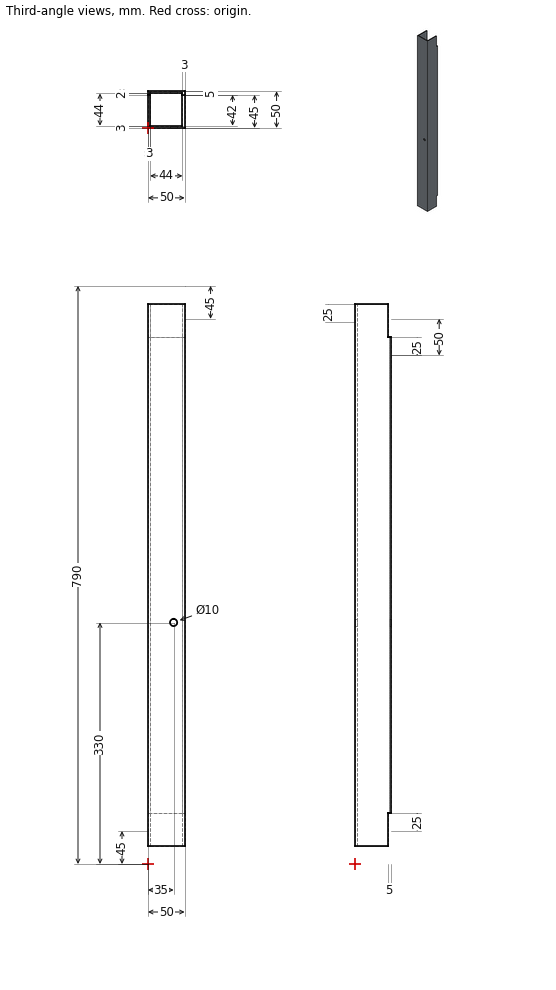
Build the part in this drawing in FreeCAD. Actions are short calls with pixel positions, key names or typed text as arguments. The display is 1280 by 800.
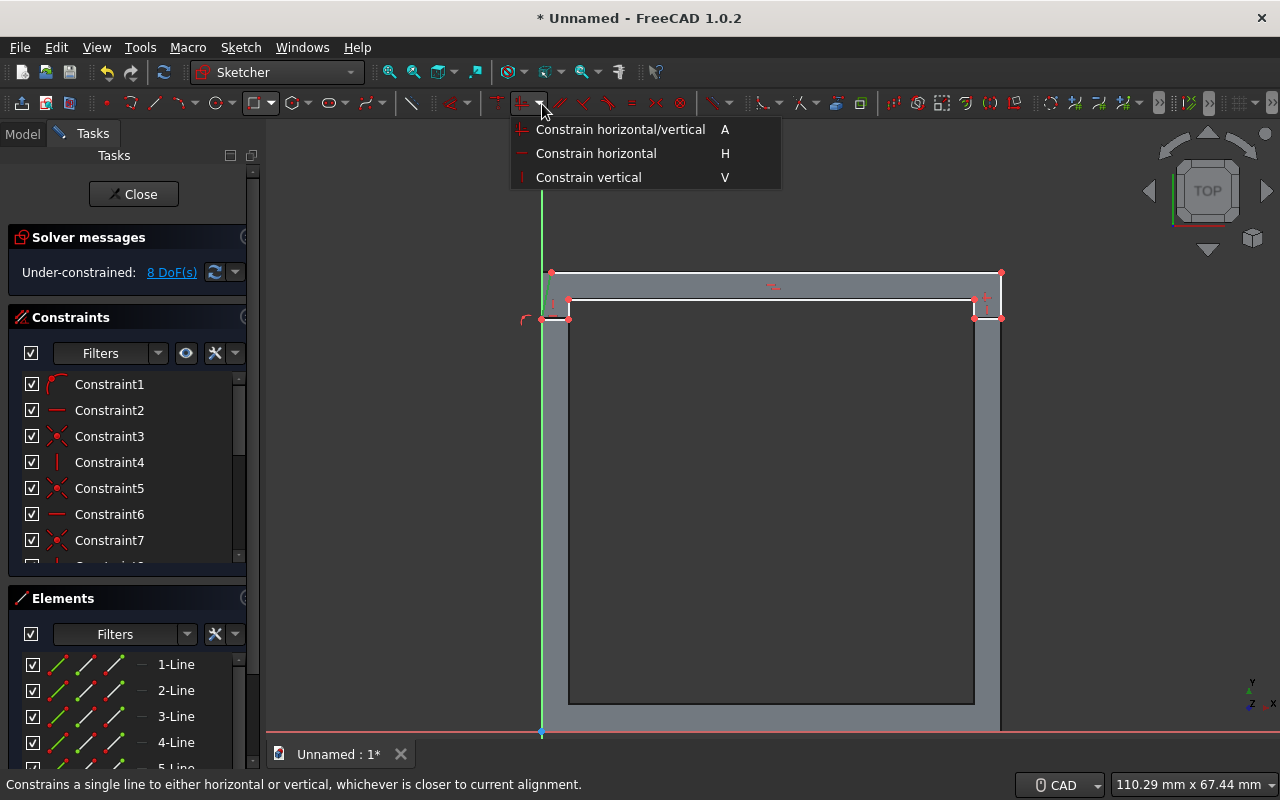
click(646, 177)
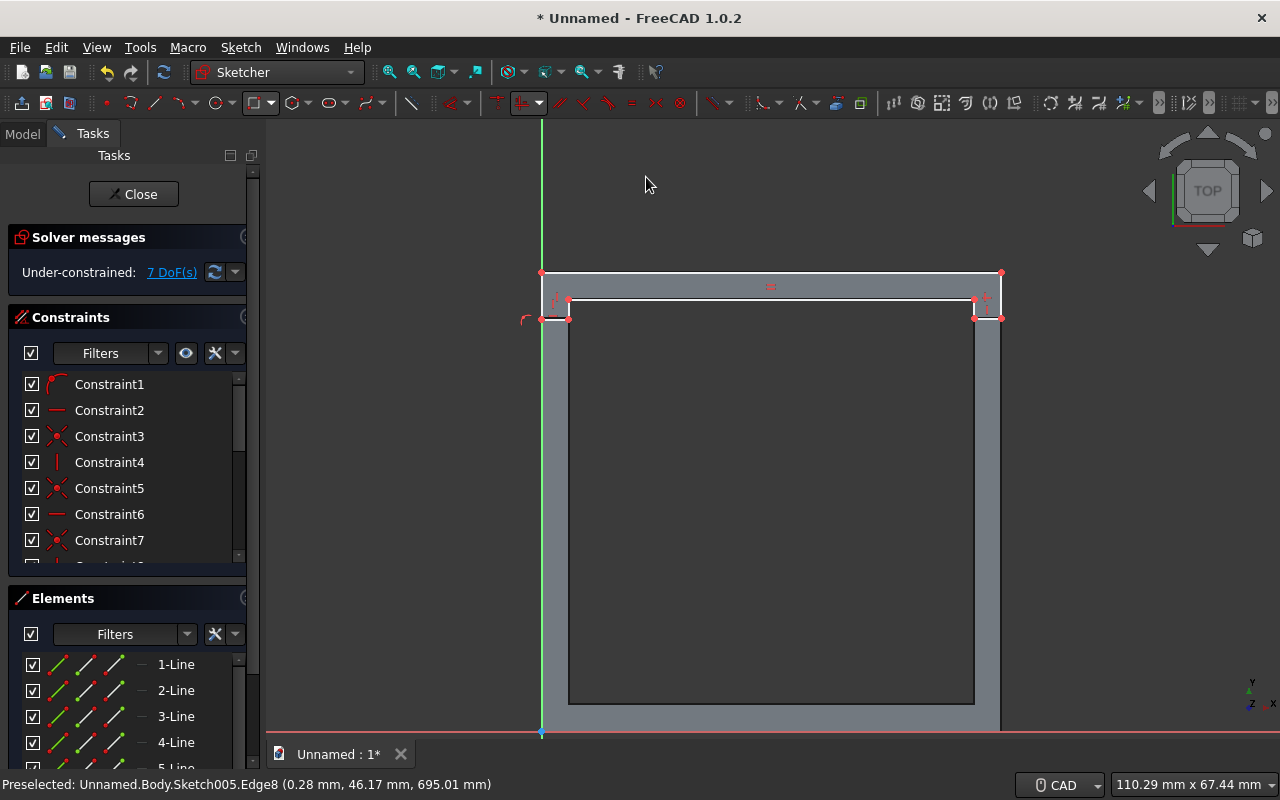
click(450, 104)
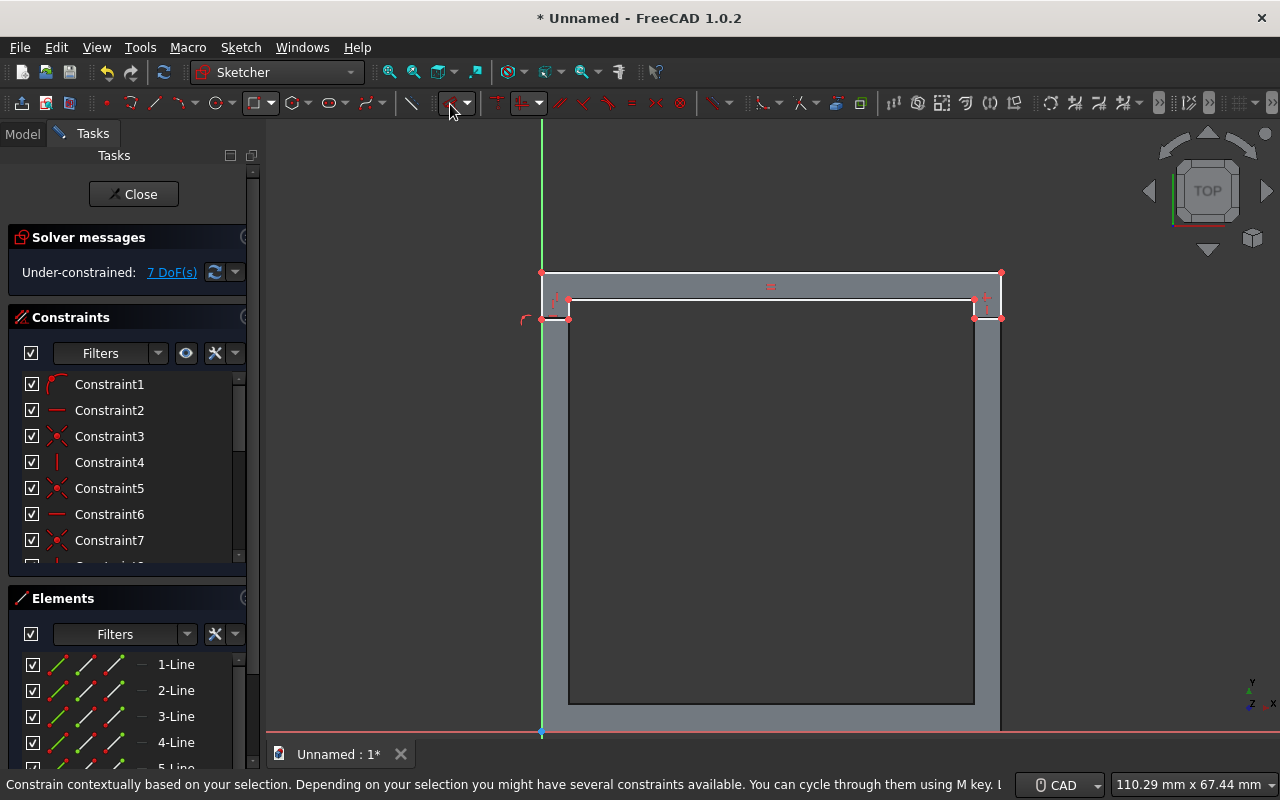
scroll(552, 320, up, 2)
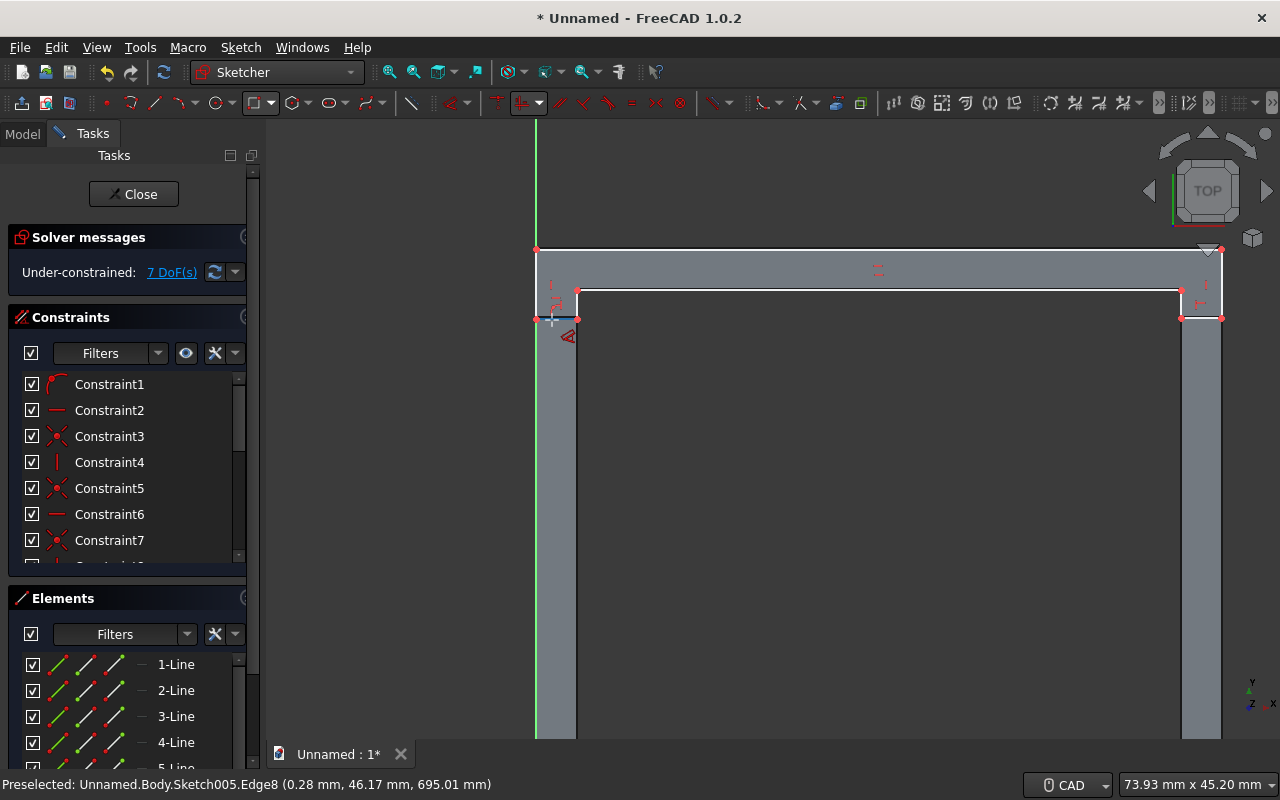
click(553, 319)
click(557, 285)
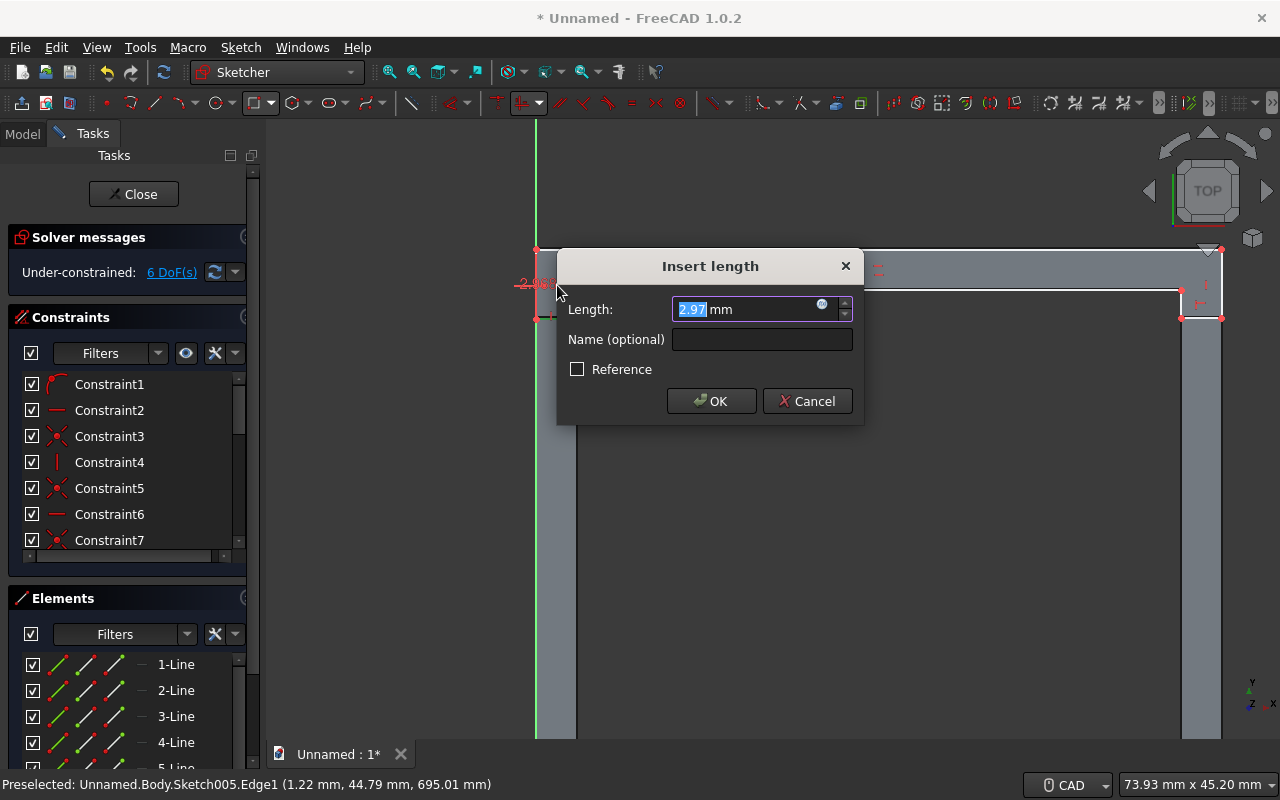
text(3)
key(Return)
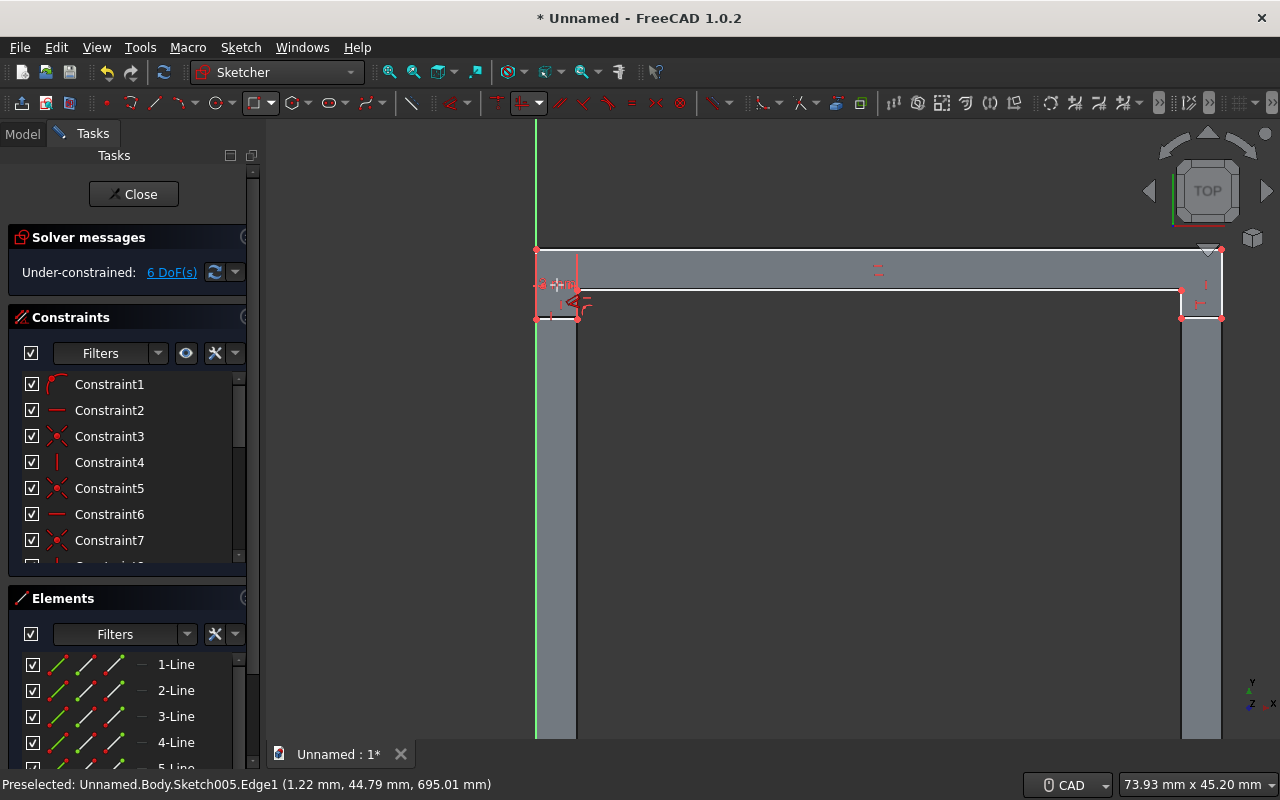
scroll(577, 308, up, 2)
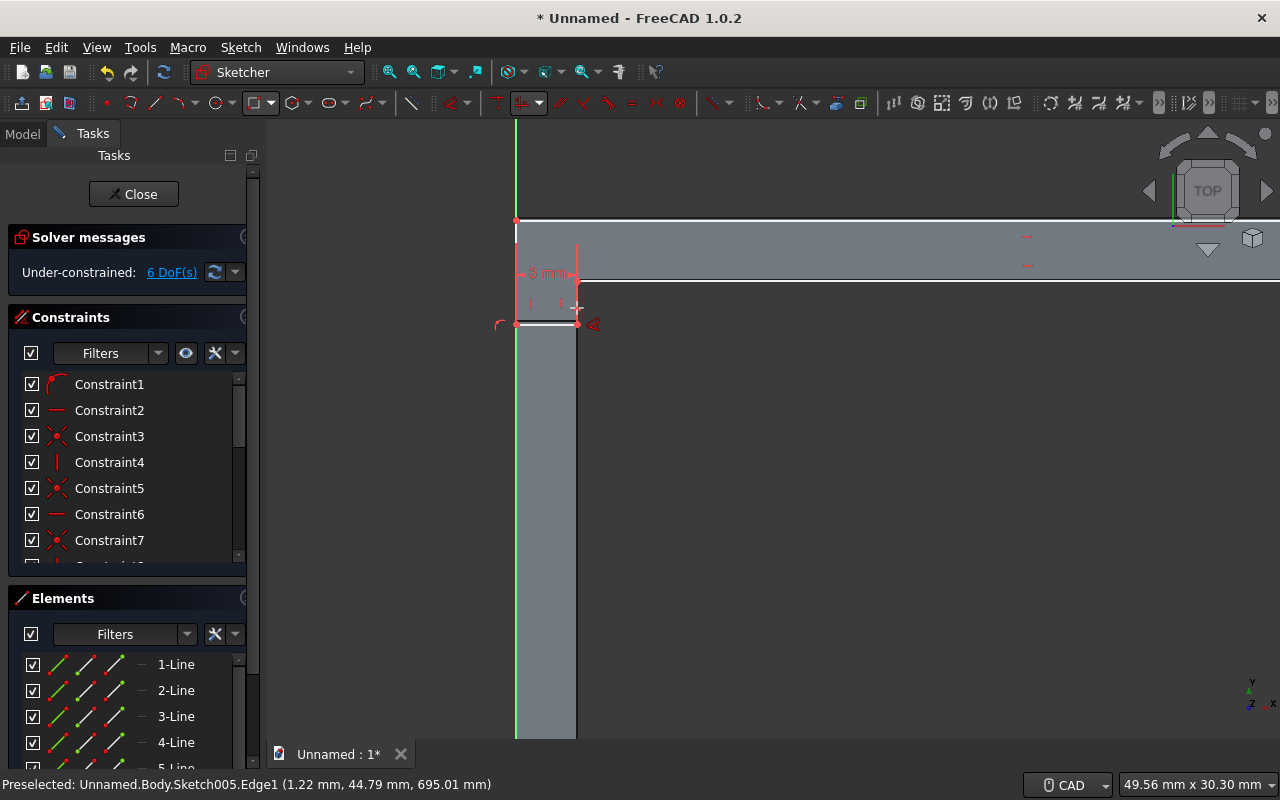
click(577, 307)
click(543, 303)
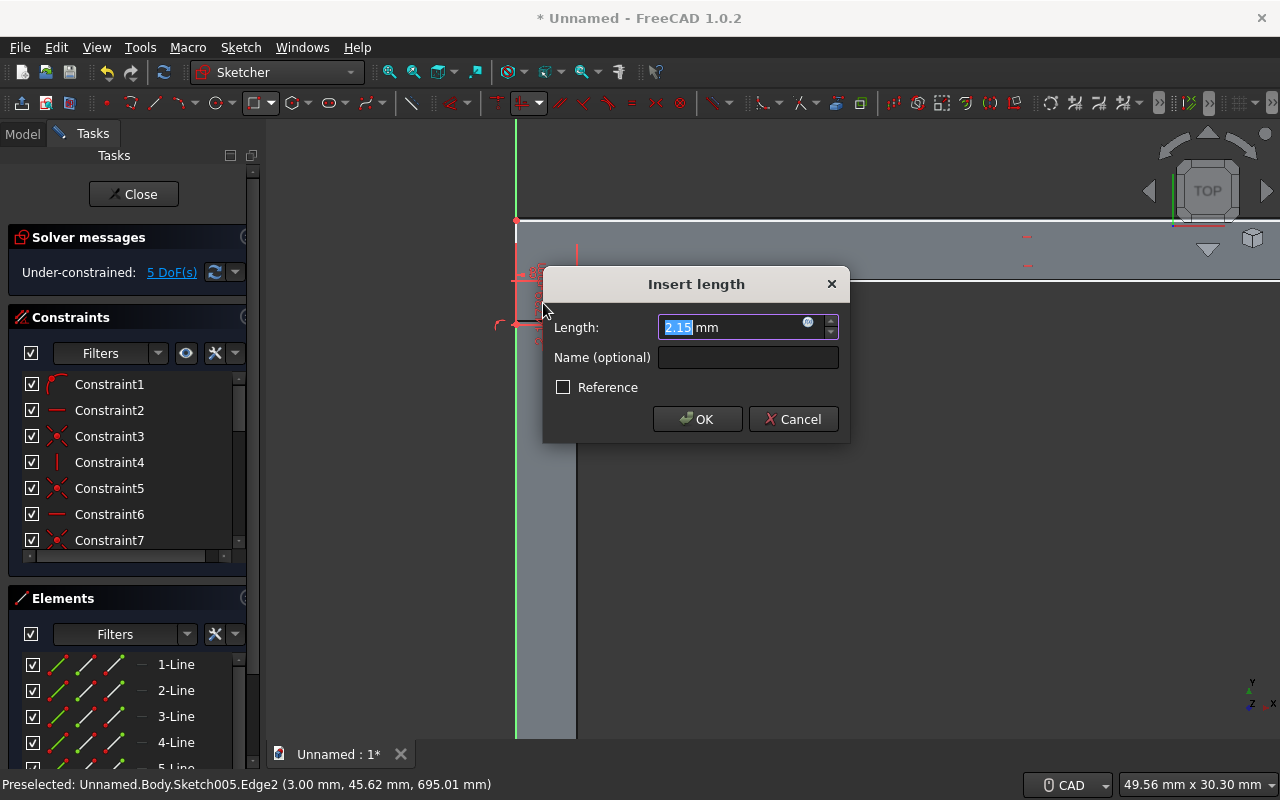
text(2)
key(Return)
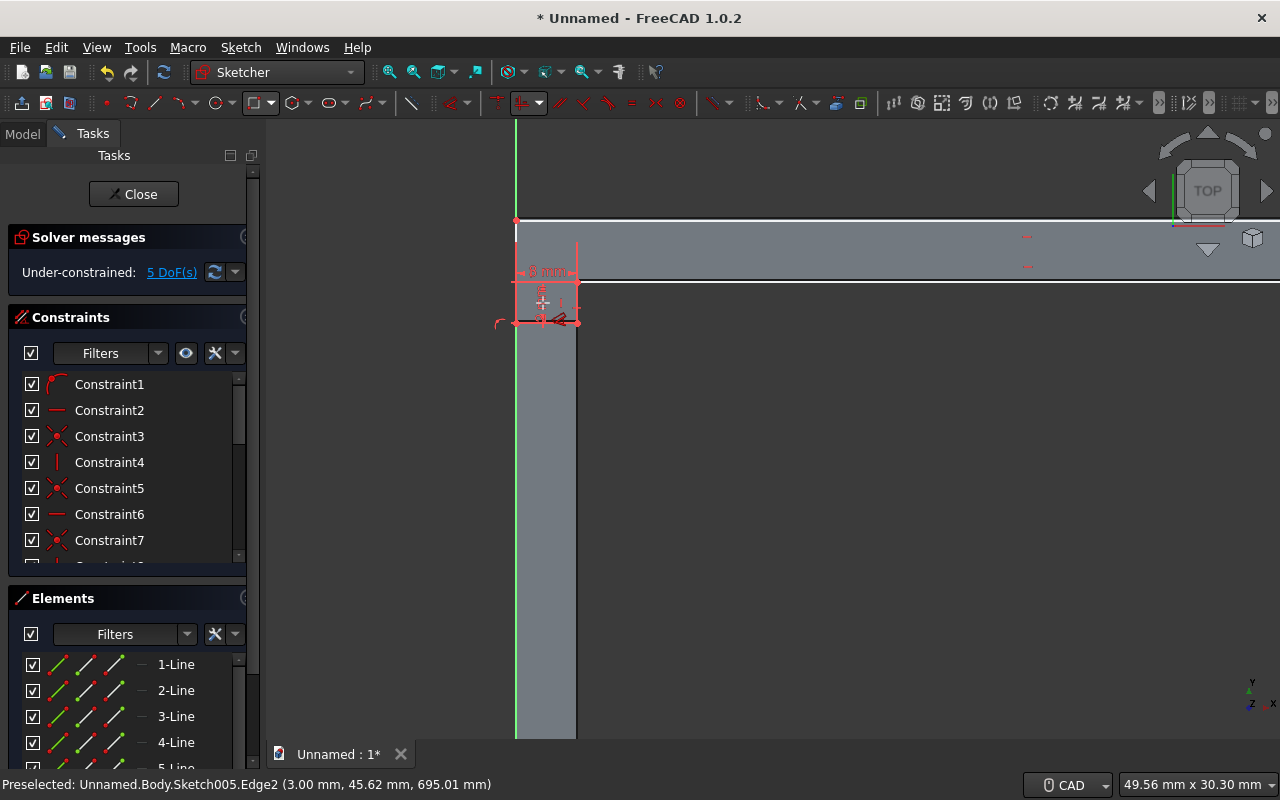
scroll(516, 254, down, 5)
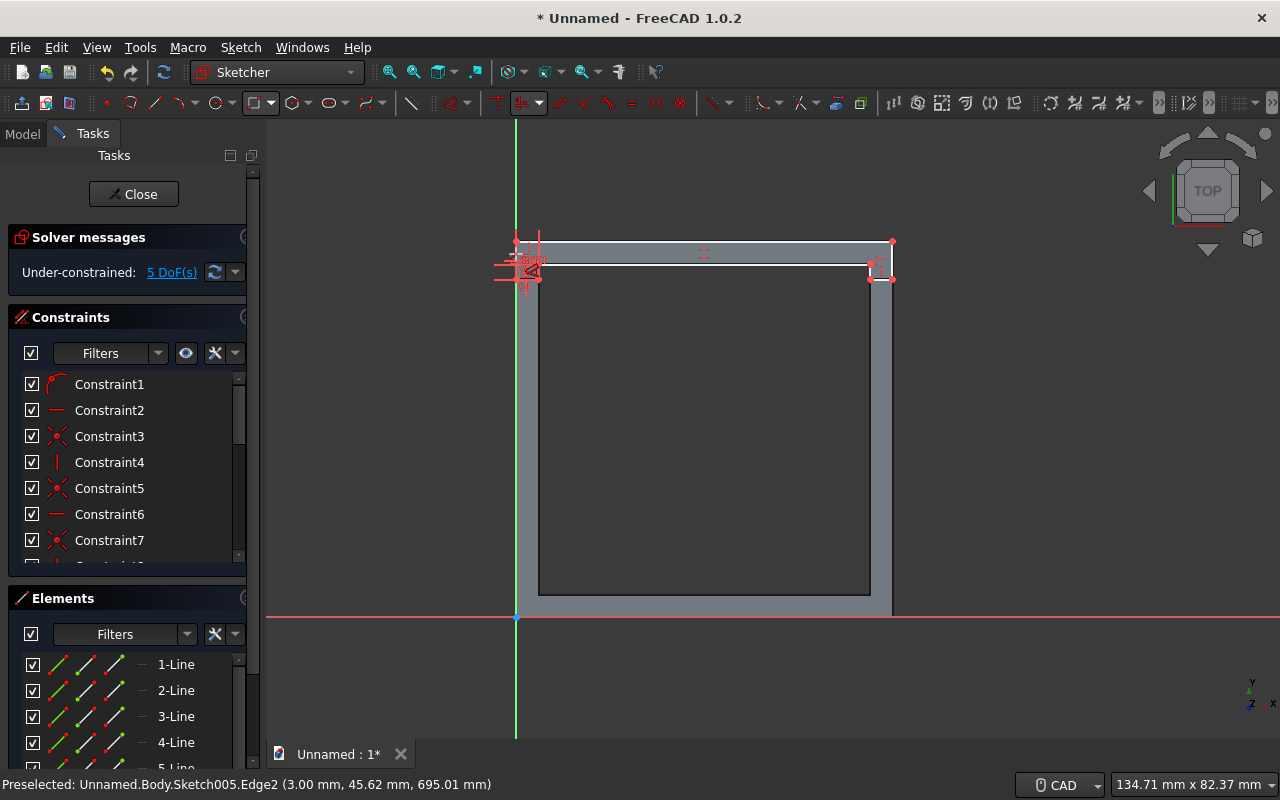
scroll(870, 269, up, 6)